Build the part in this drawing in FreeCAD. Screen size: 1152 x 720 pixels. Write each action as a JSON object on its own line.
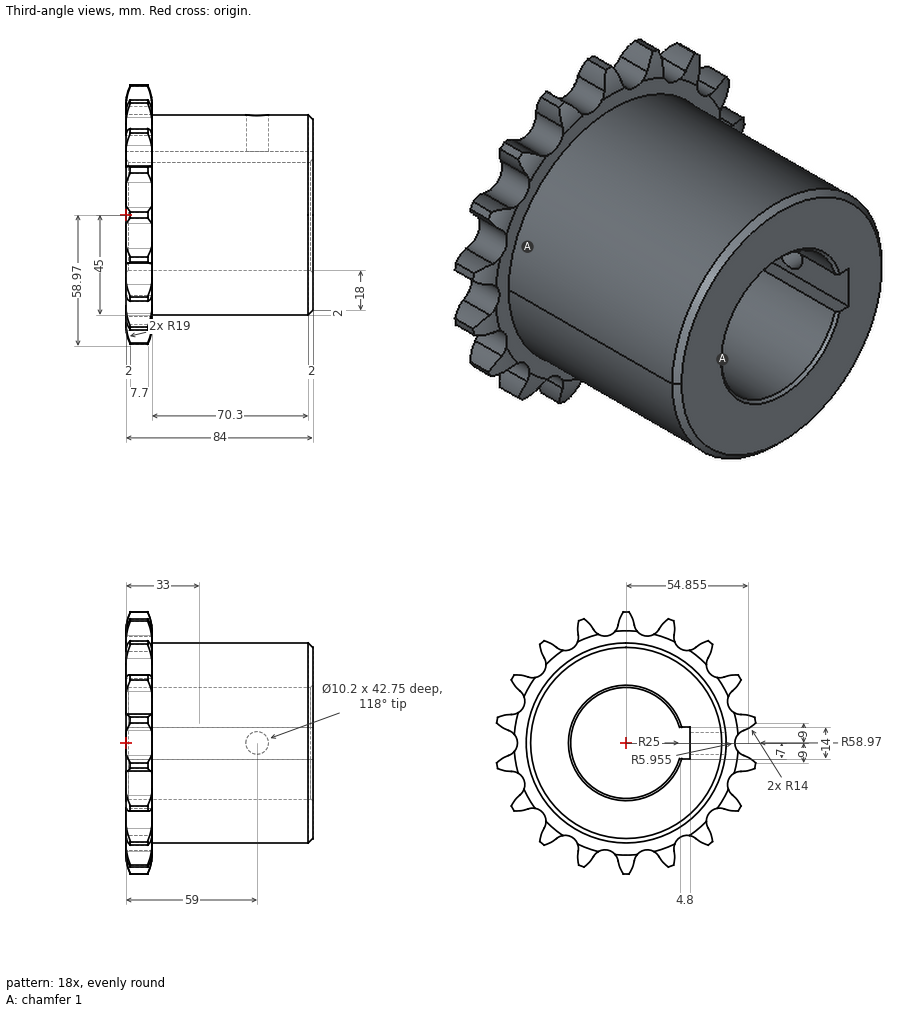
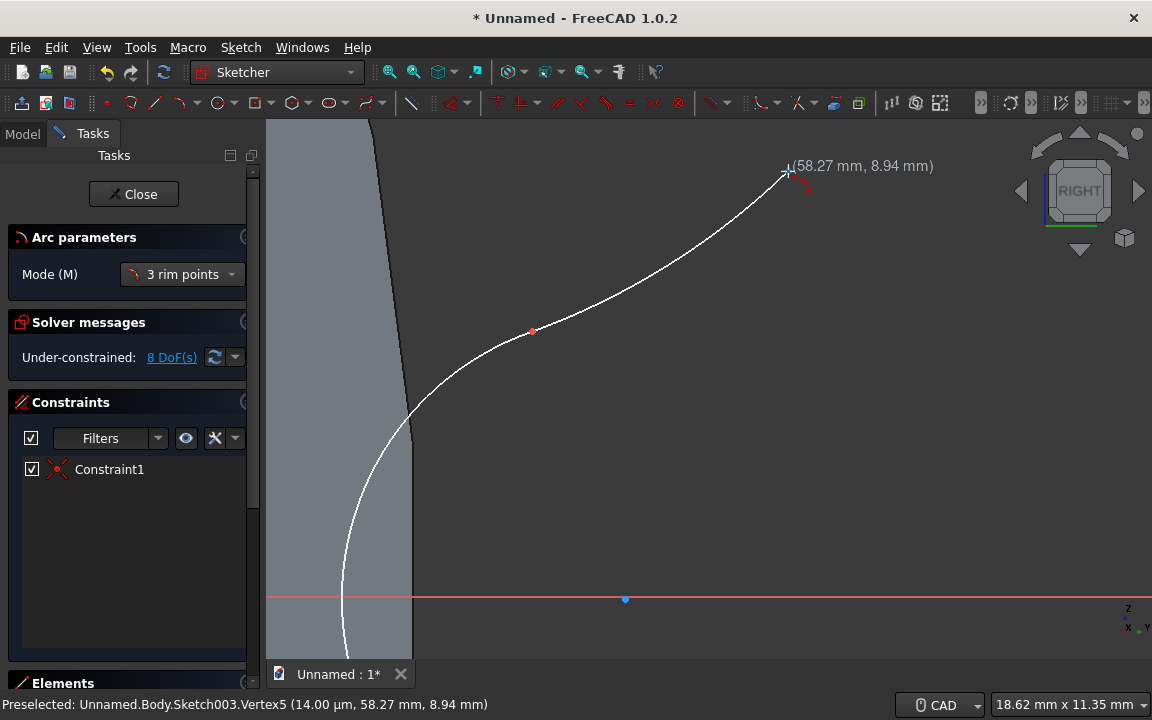
{"action": "scroll", "coordinate": [675, 268], "scroll_direction": "down", "scroll_amount": 5}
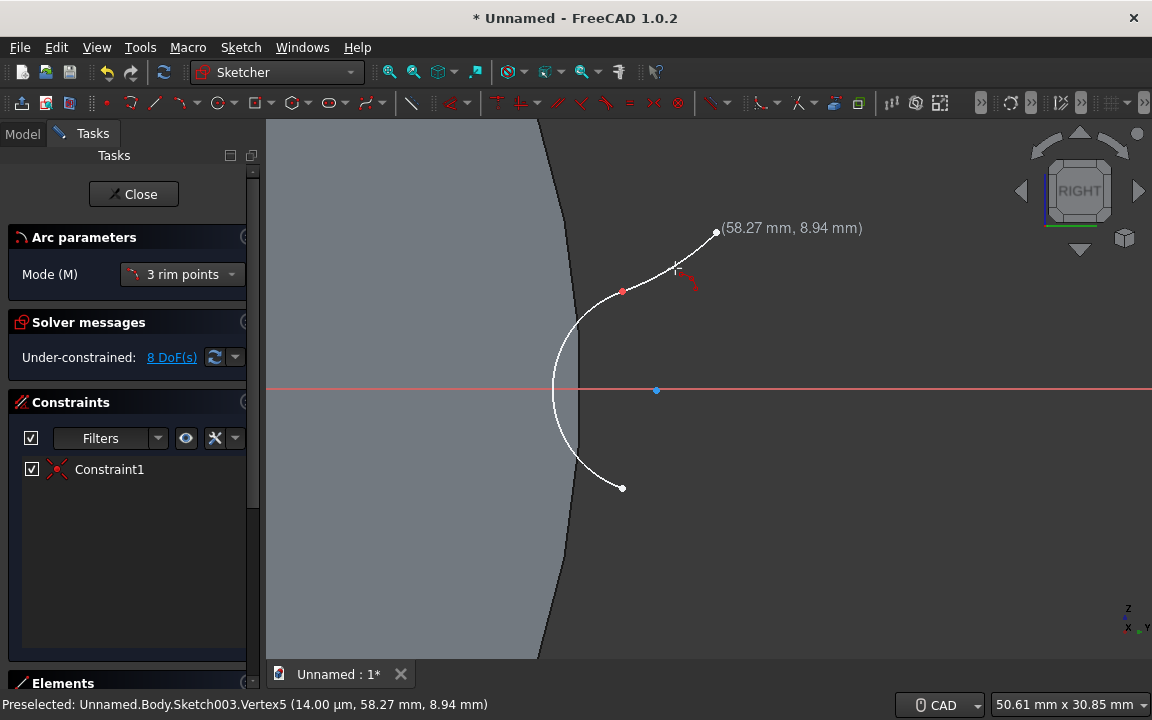
{"action": "left_click", "coordinate": [717, 547]}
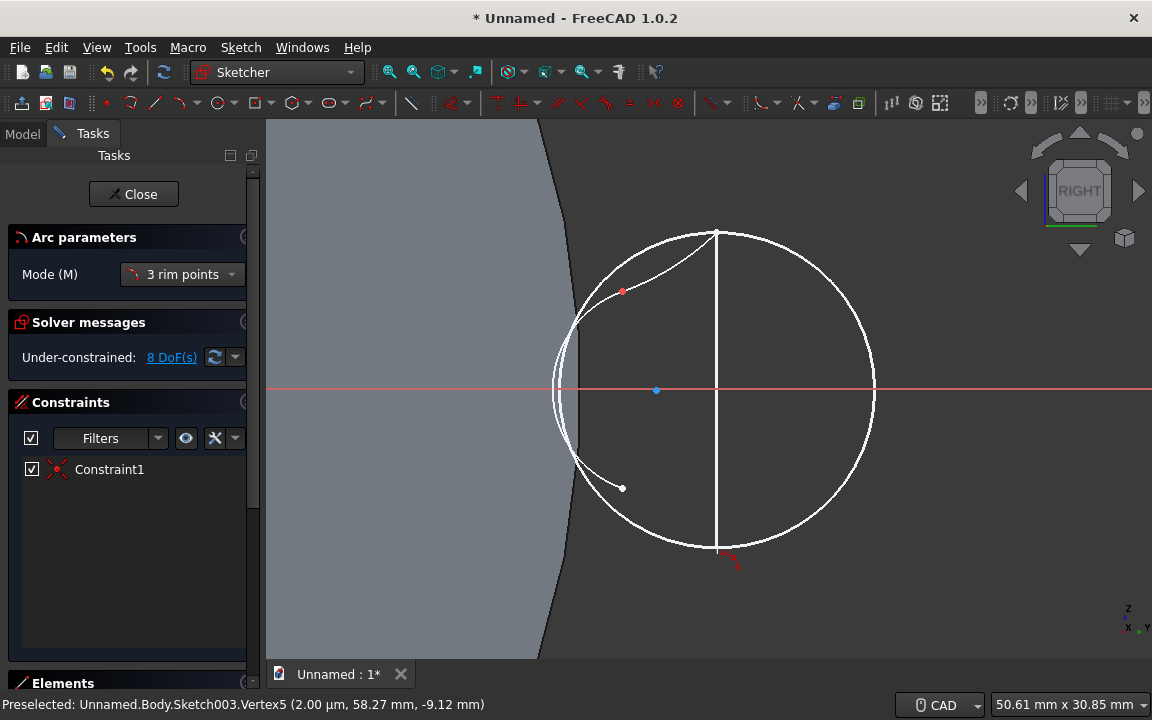
{"action": "scroll", "coordinate": [729, 421], "scroll_direction": "up", "scroll_amount": 2}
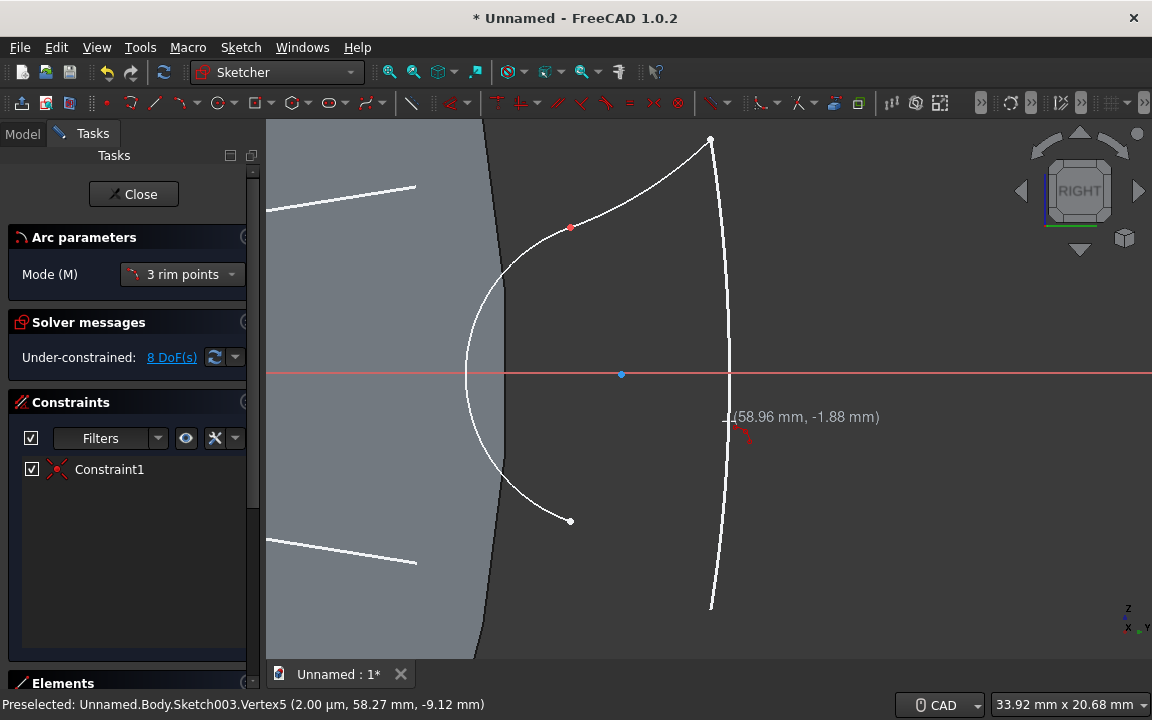
{"action": "left_click", "coordinate": [728, 420]}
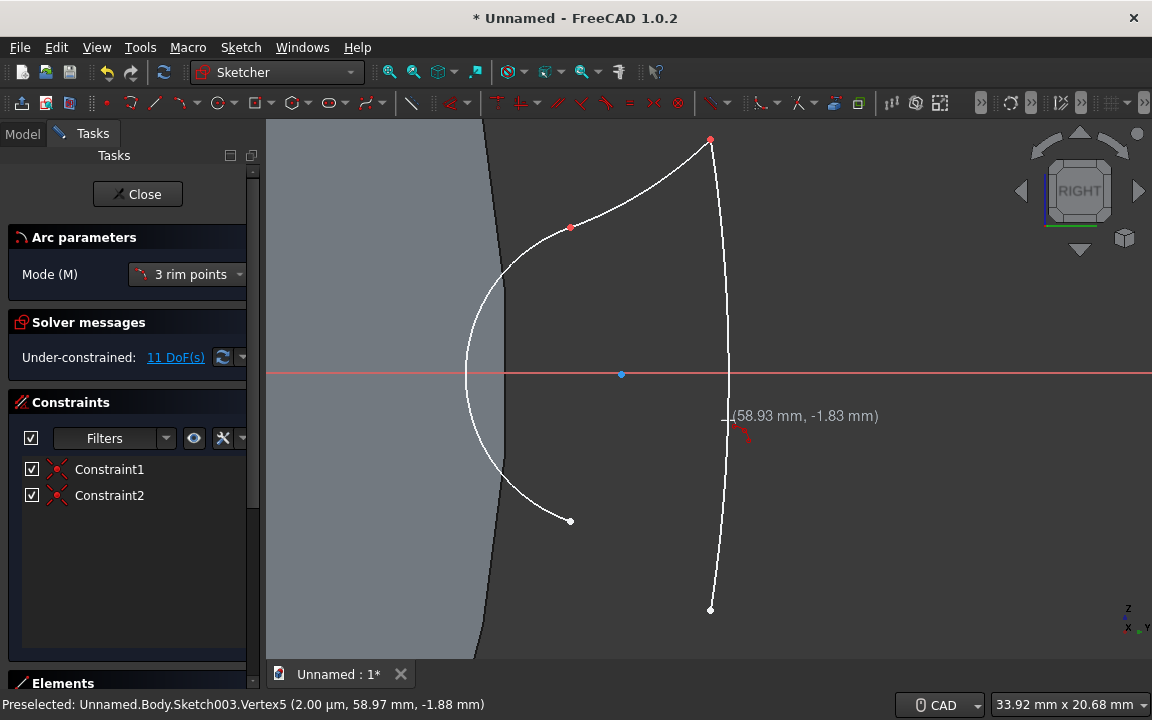
{"action": "left_click", "coordinate": [711, 610]}
{"action": "left_click", "coordinate": [570, 521]}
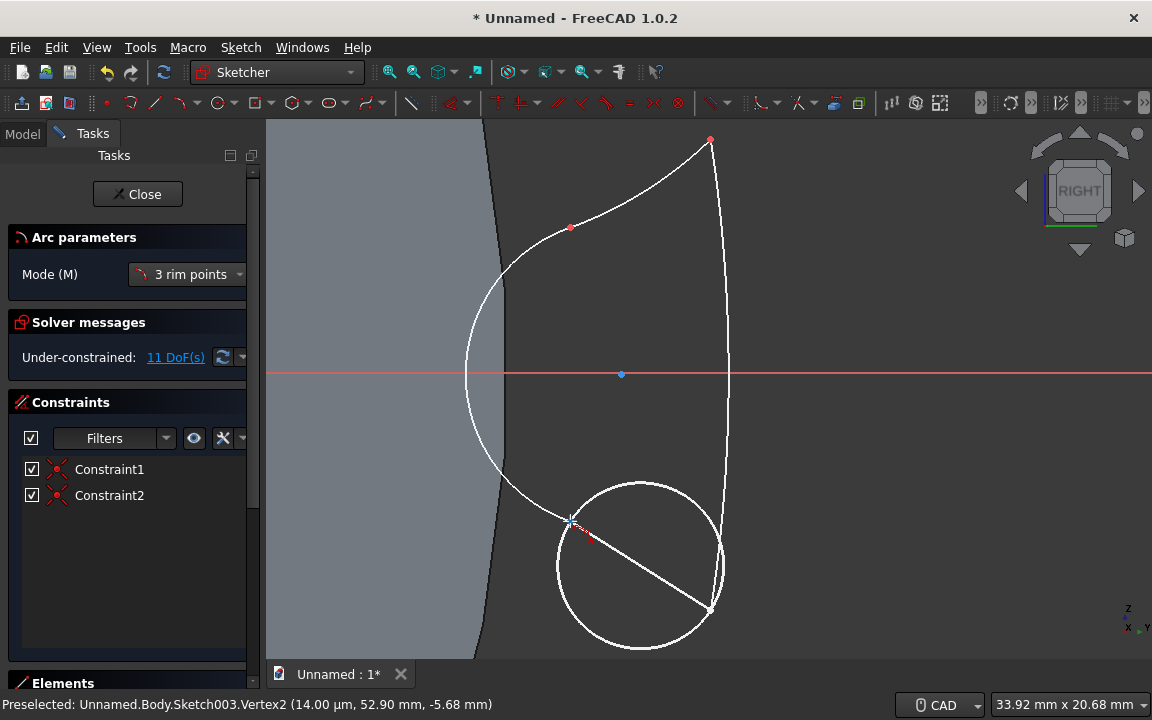
{"action": "scroll", "coordinate": [646, 556], "scroll_direction": "up", "scroll_amount": 3}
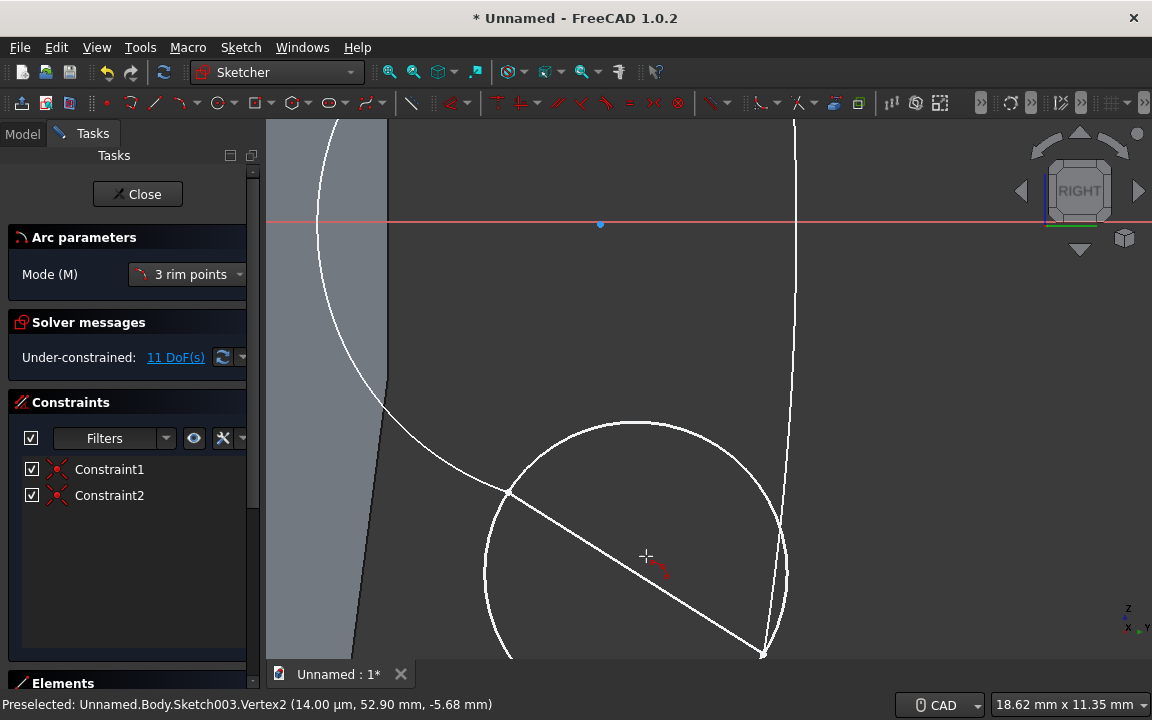
{"action": "left_click", "coordinate": [646, 556]}
{"action": "key", "text": "Escape"}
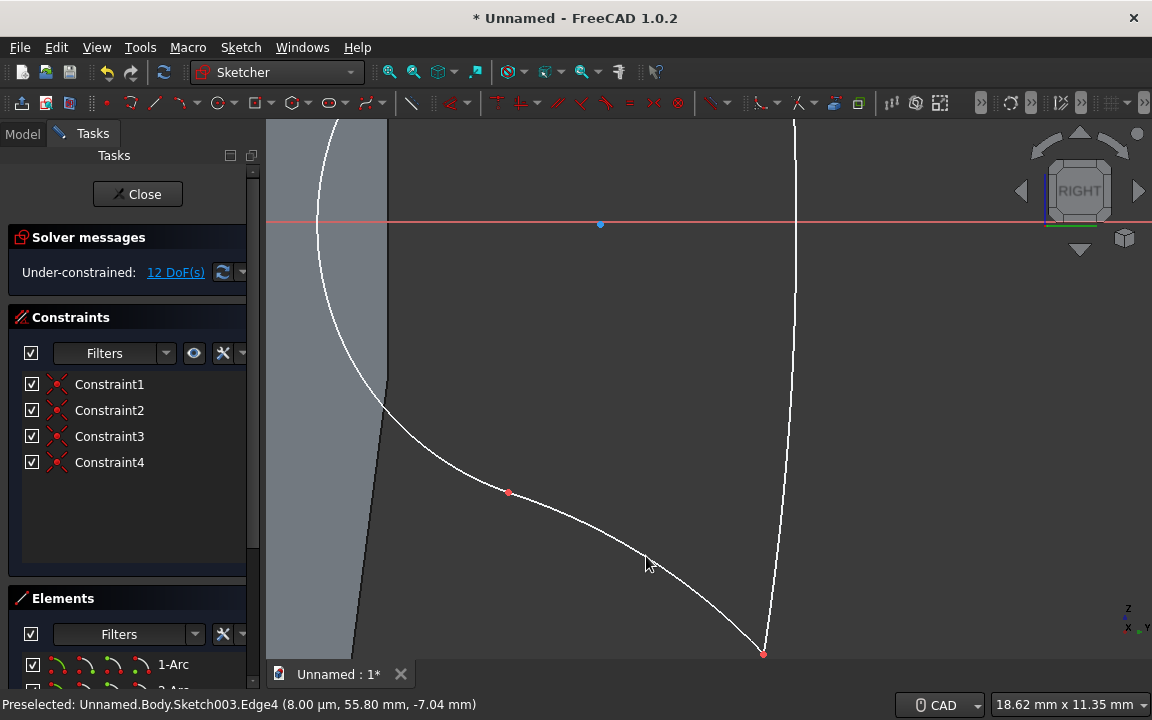
{"action": "left_click", "coordinate": [351, 359]}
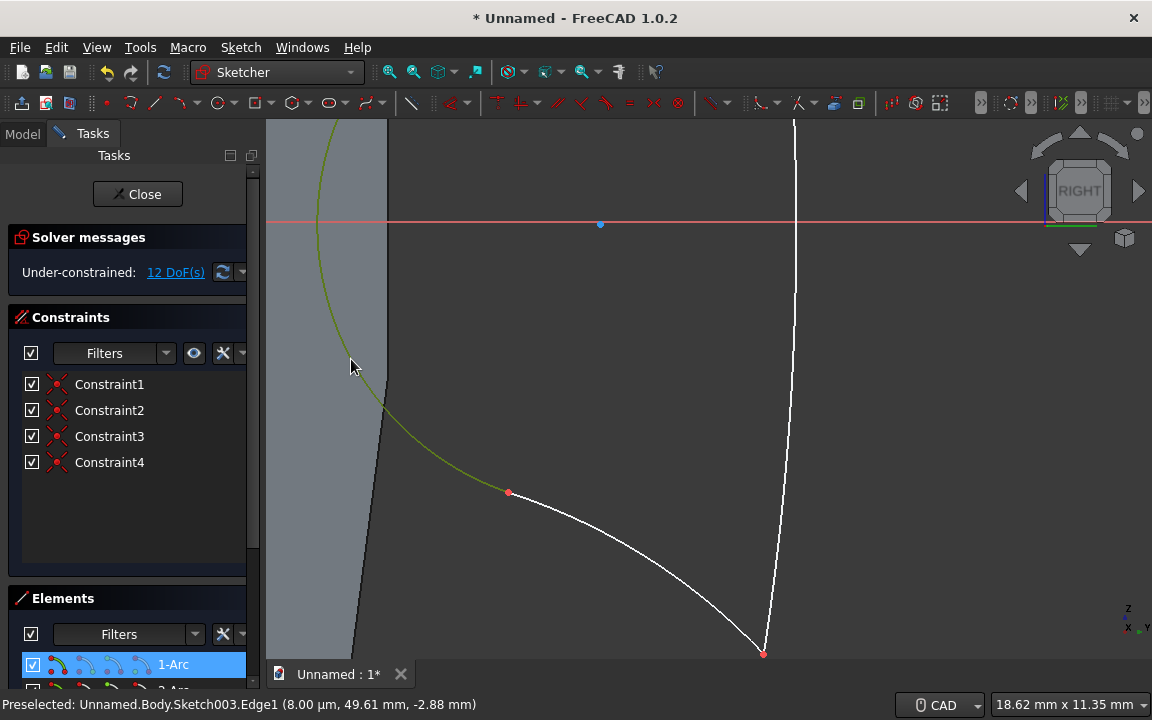
{"action": "scroll", "coordinate": [689, 486], "scroll_direction": "down", "scroll_amount": 5}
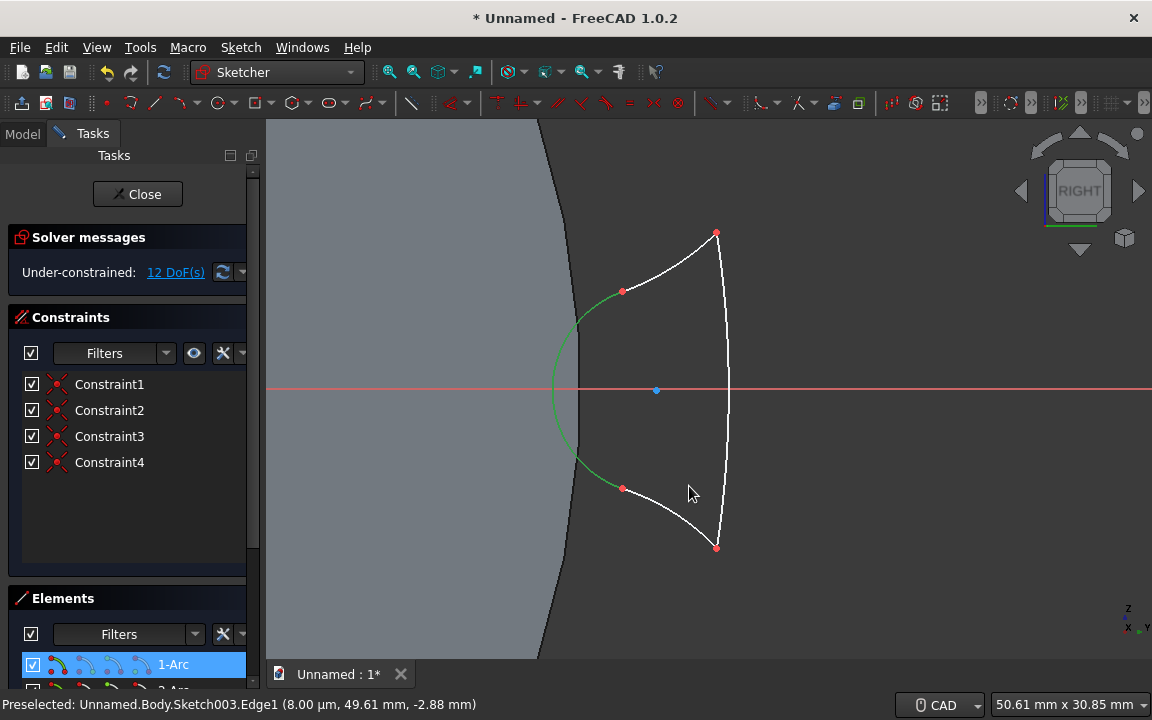
{"action": "left_click", "coordinate": [653, 278]}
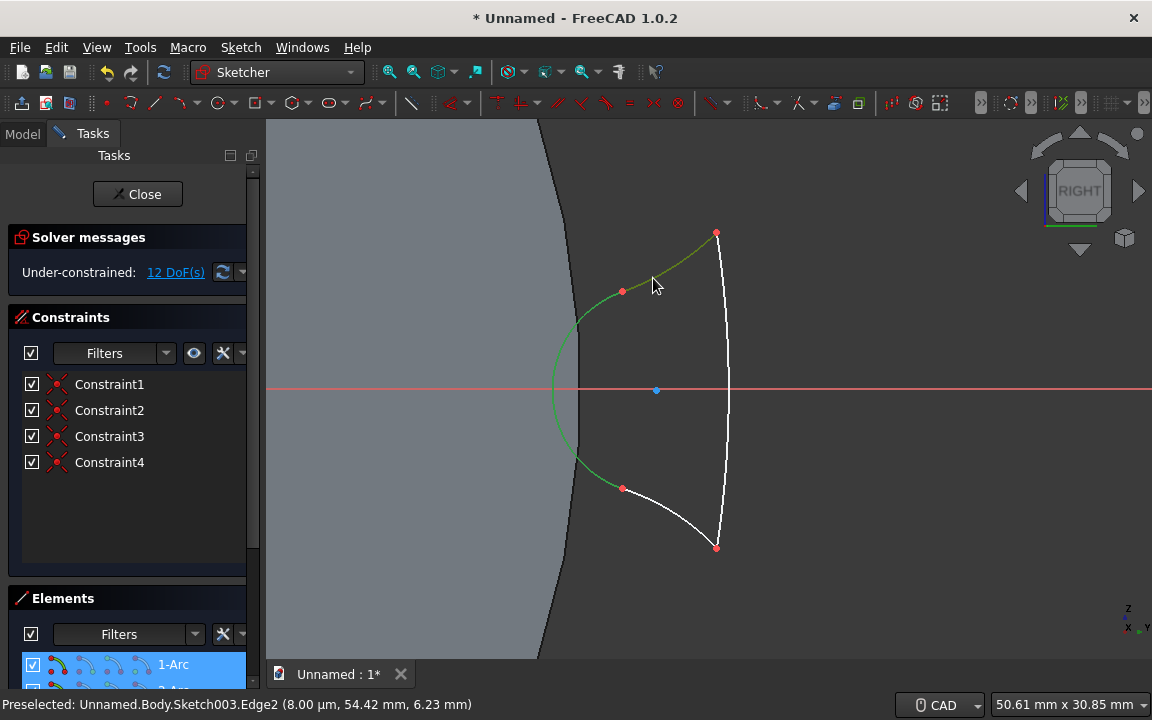
{"action": "left_click", "coordinate": [606, 104]}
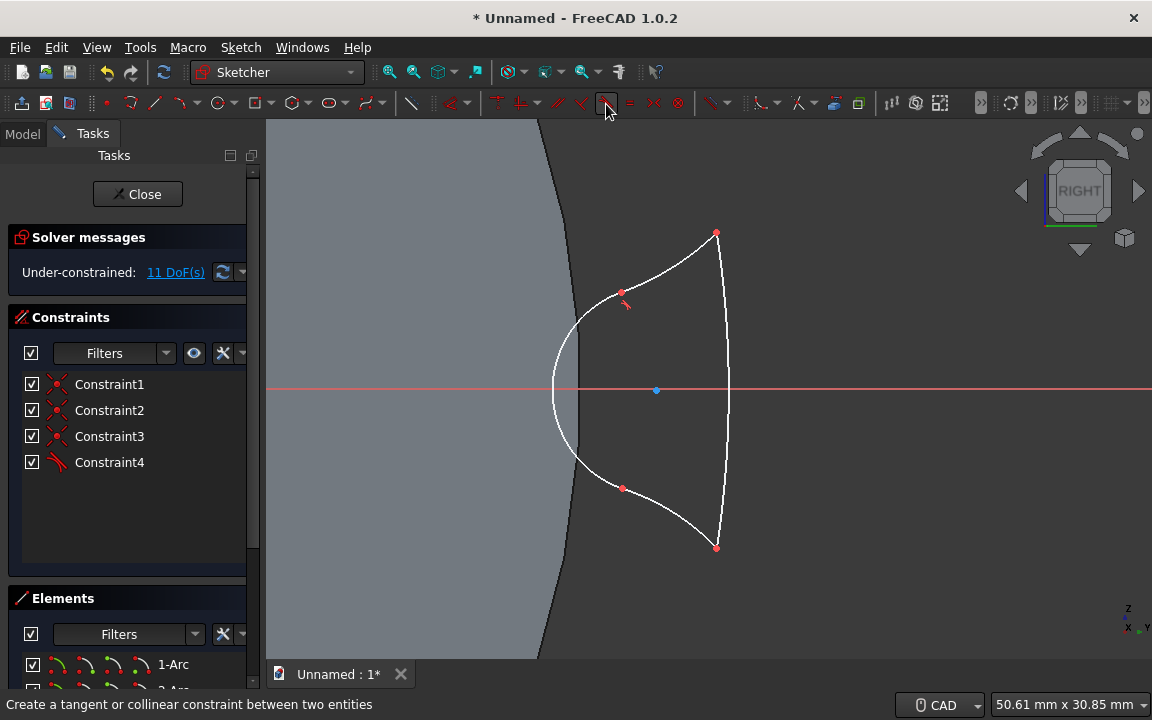
{"action": "left_click", "coordinate": [565, 342]}